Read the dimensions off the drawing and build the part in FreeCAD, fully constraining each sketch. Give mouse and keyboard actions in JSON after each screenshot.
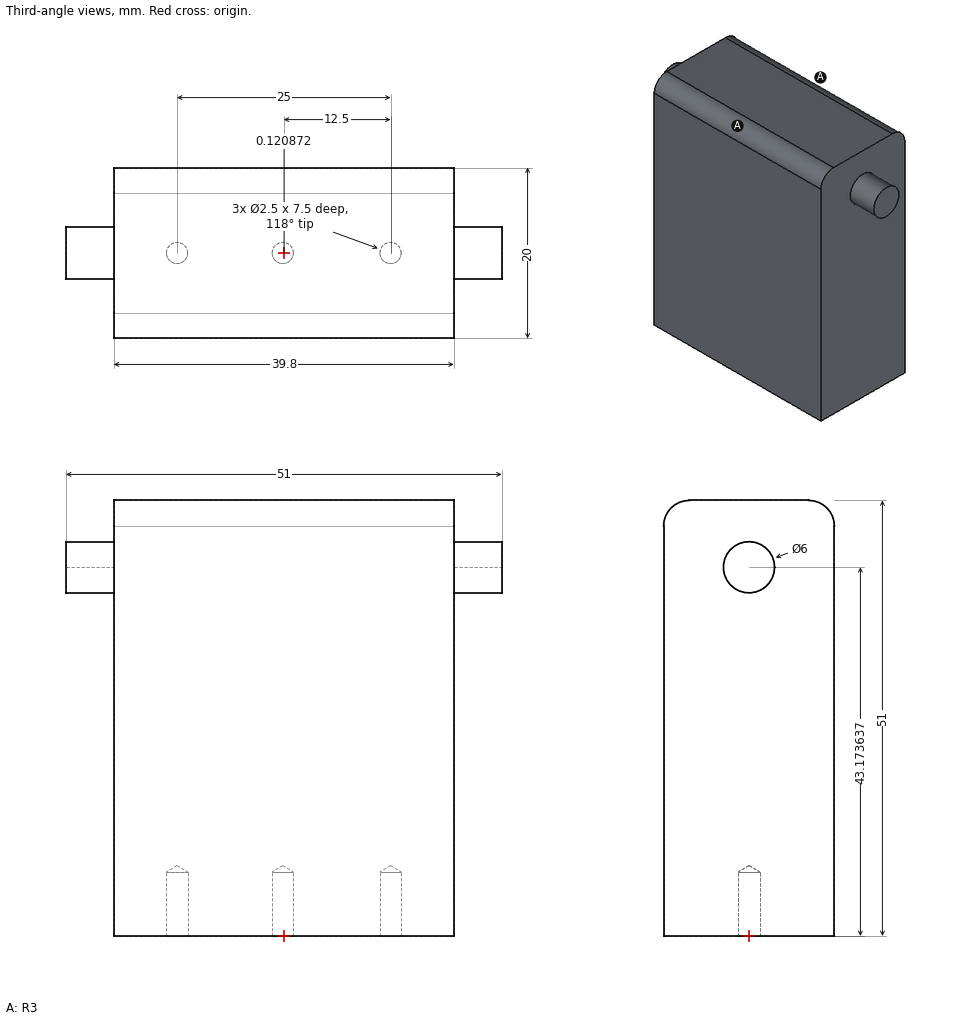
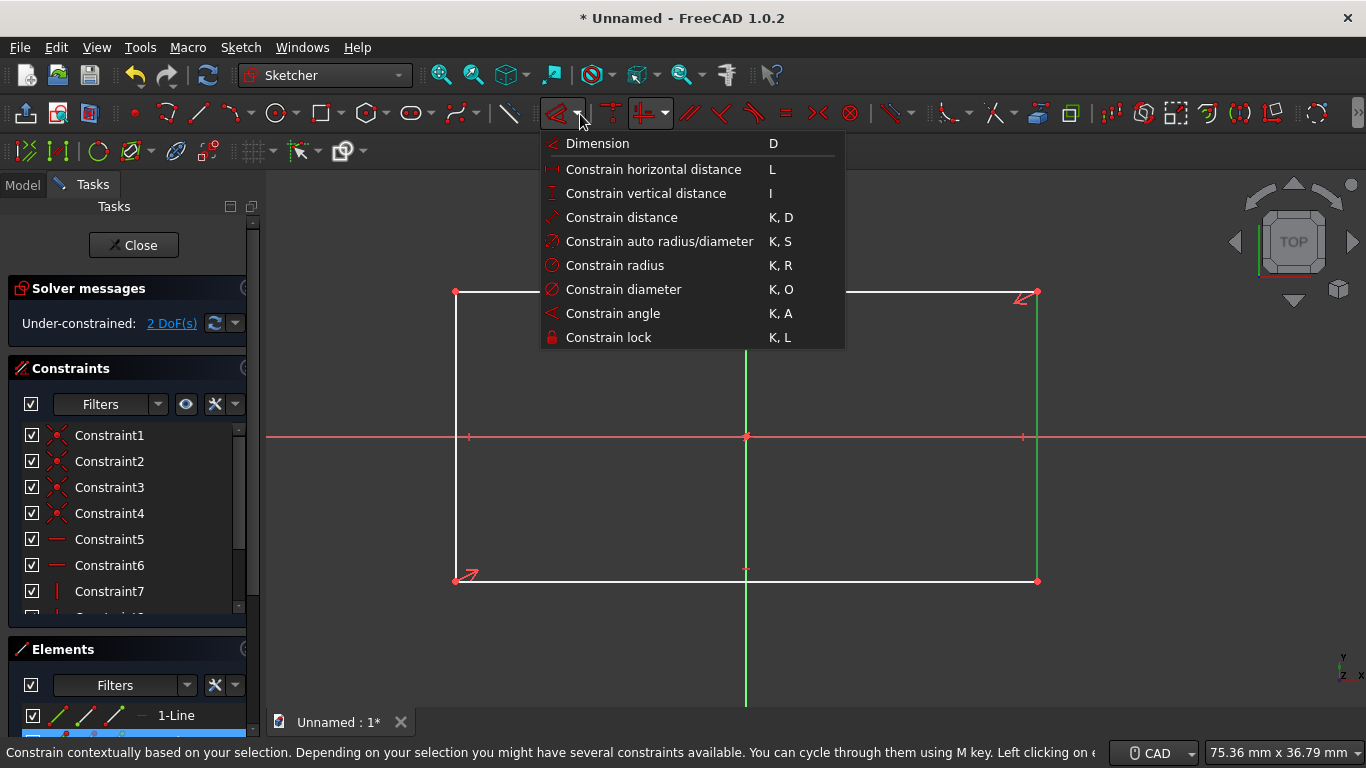
{"action": "left_click", "coordinate": [693, 193]}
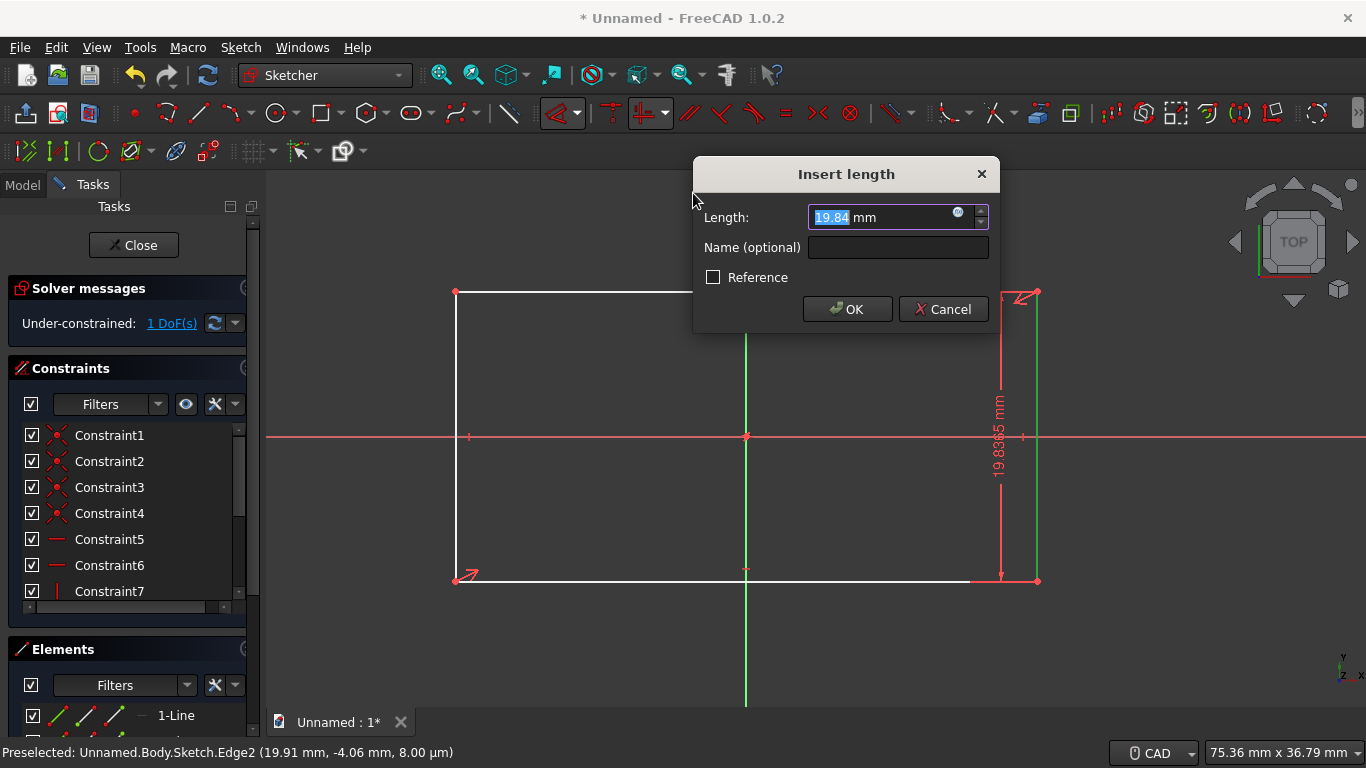
{"action": "type", "text": "20"}
{"action": "key", "text": "Return"}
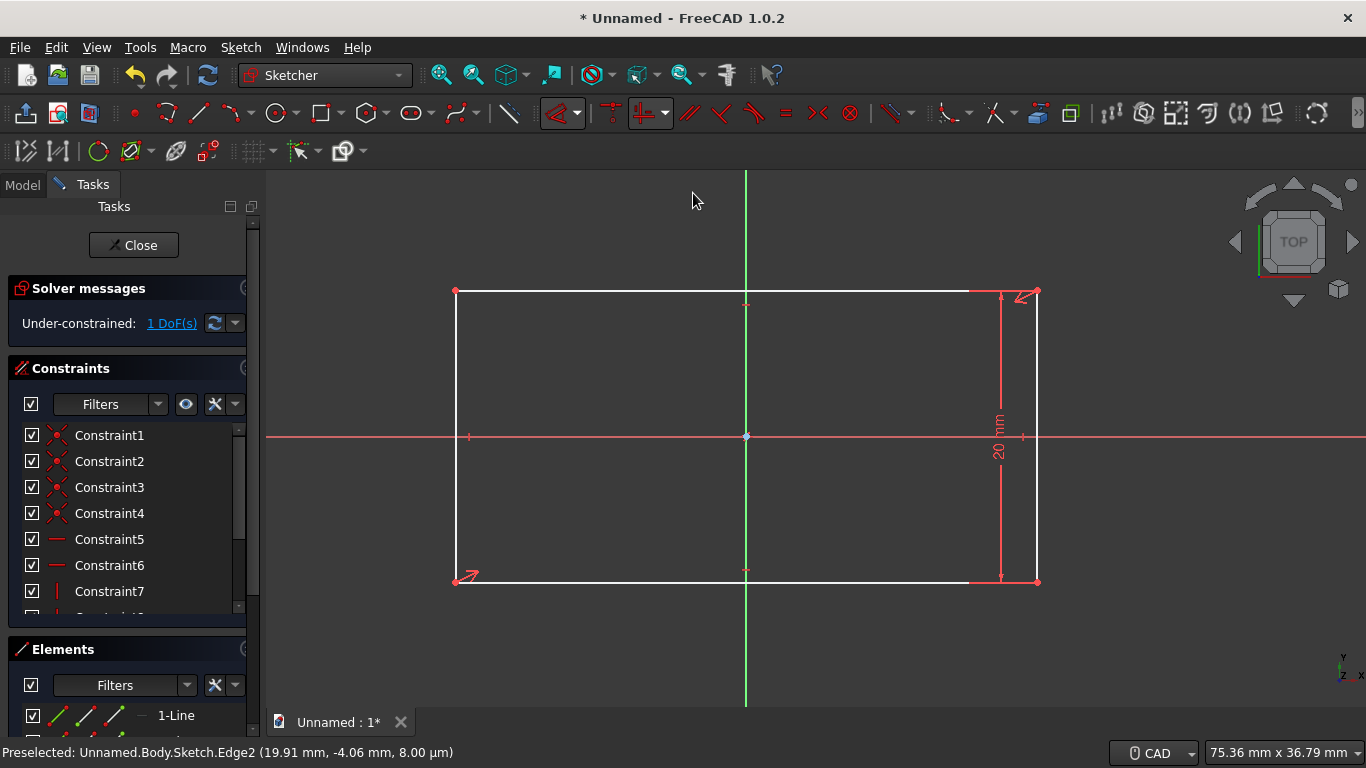
{"action": "left_click", "coordinate": [630, 583]}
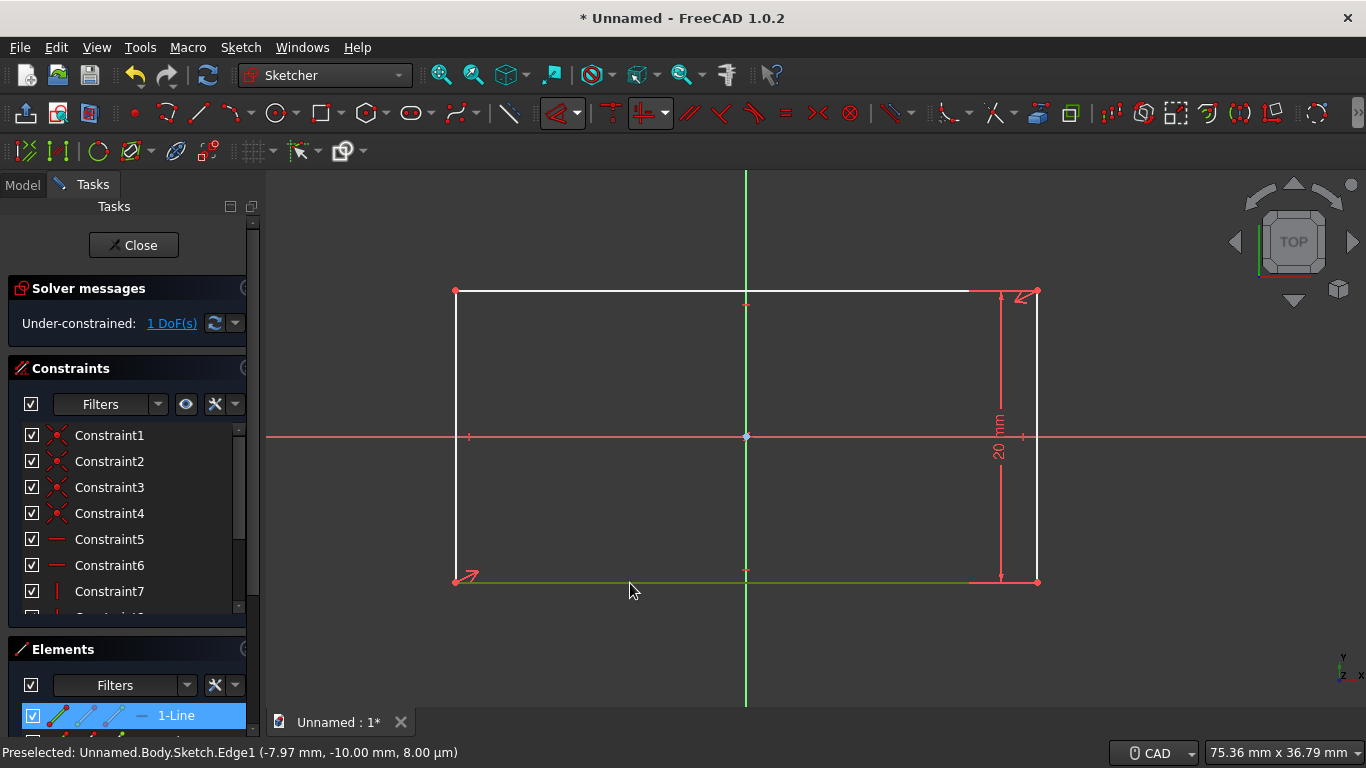
{"action": "key", "text": "l"}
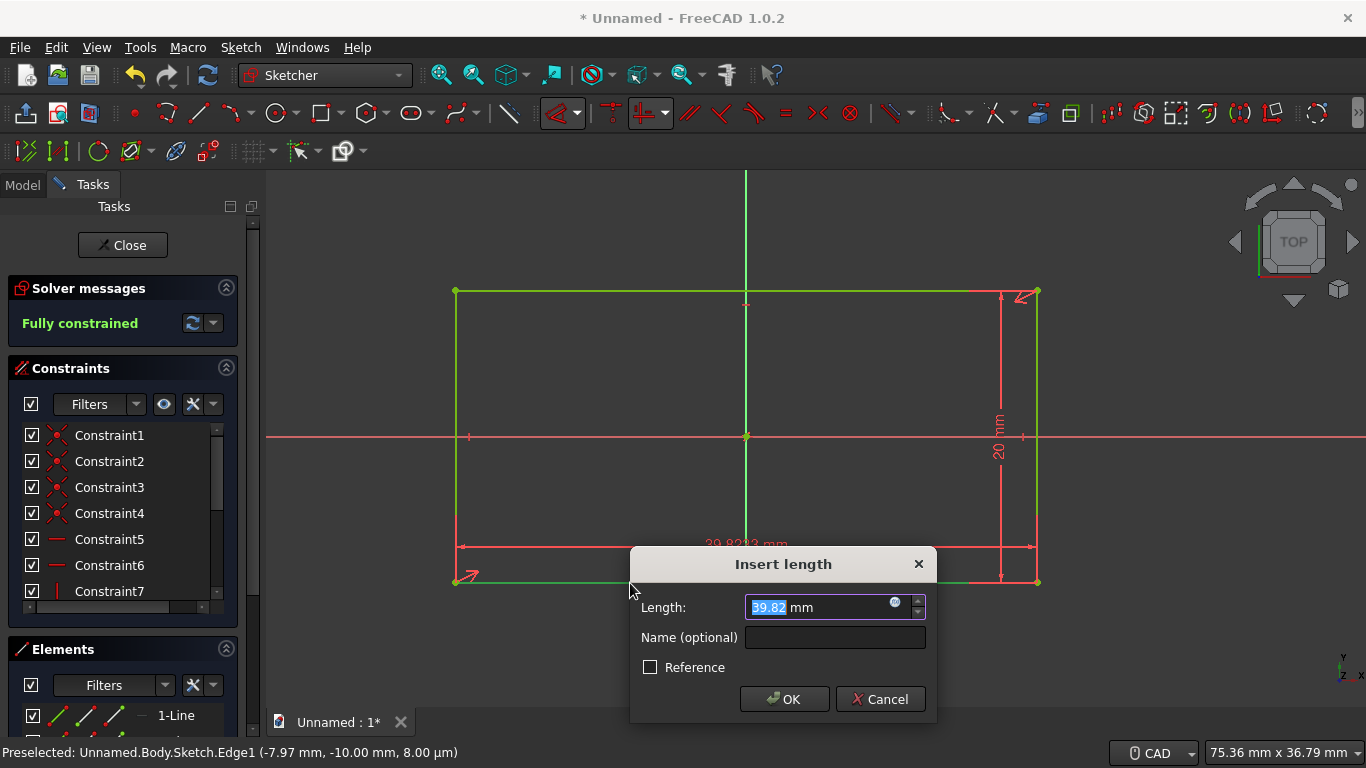
{"action": "type", "text": "39.8"}
{"action": "key", "text": "Return"}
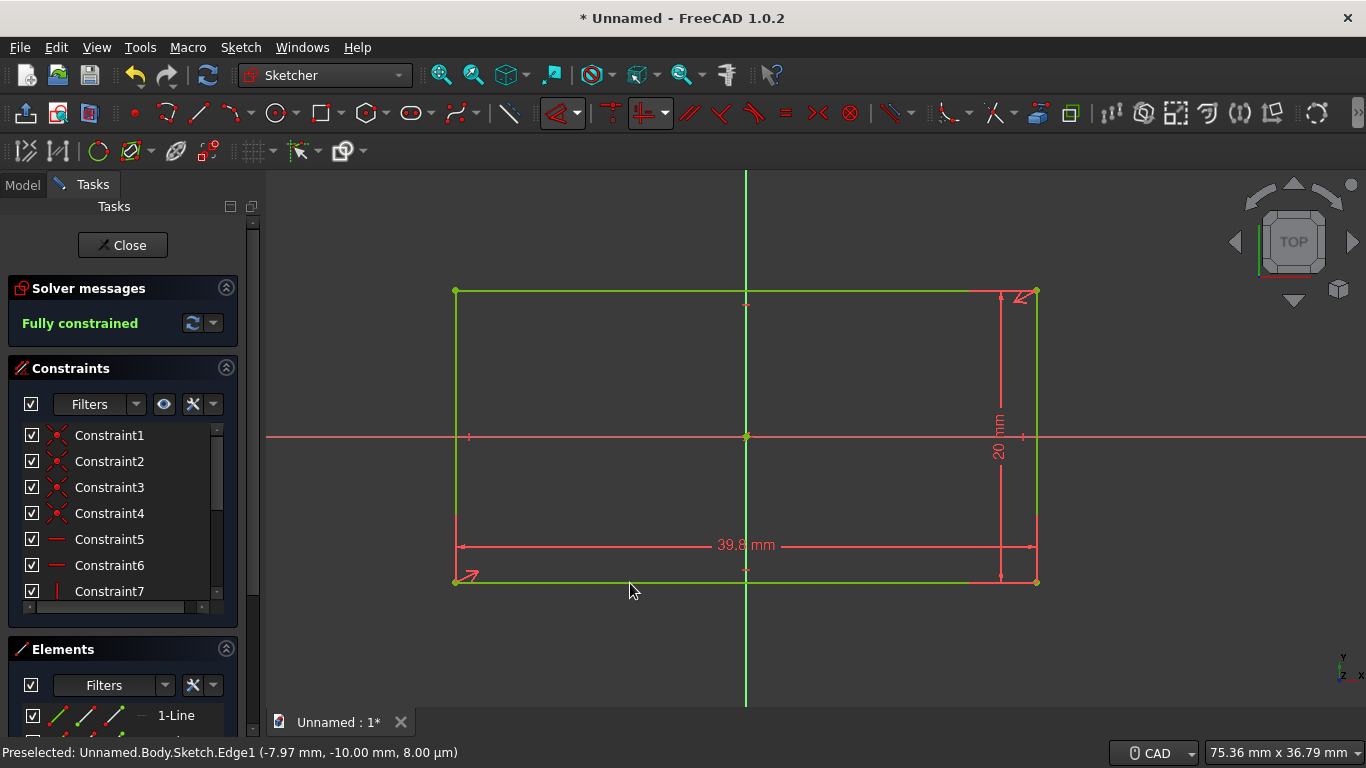
{"action": "left_click", "coordinate": [123, 245]}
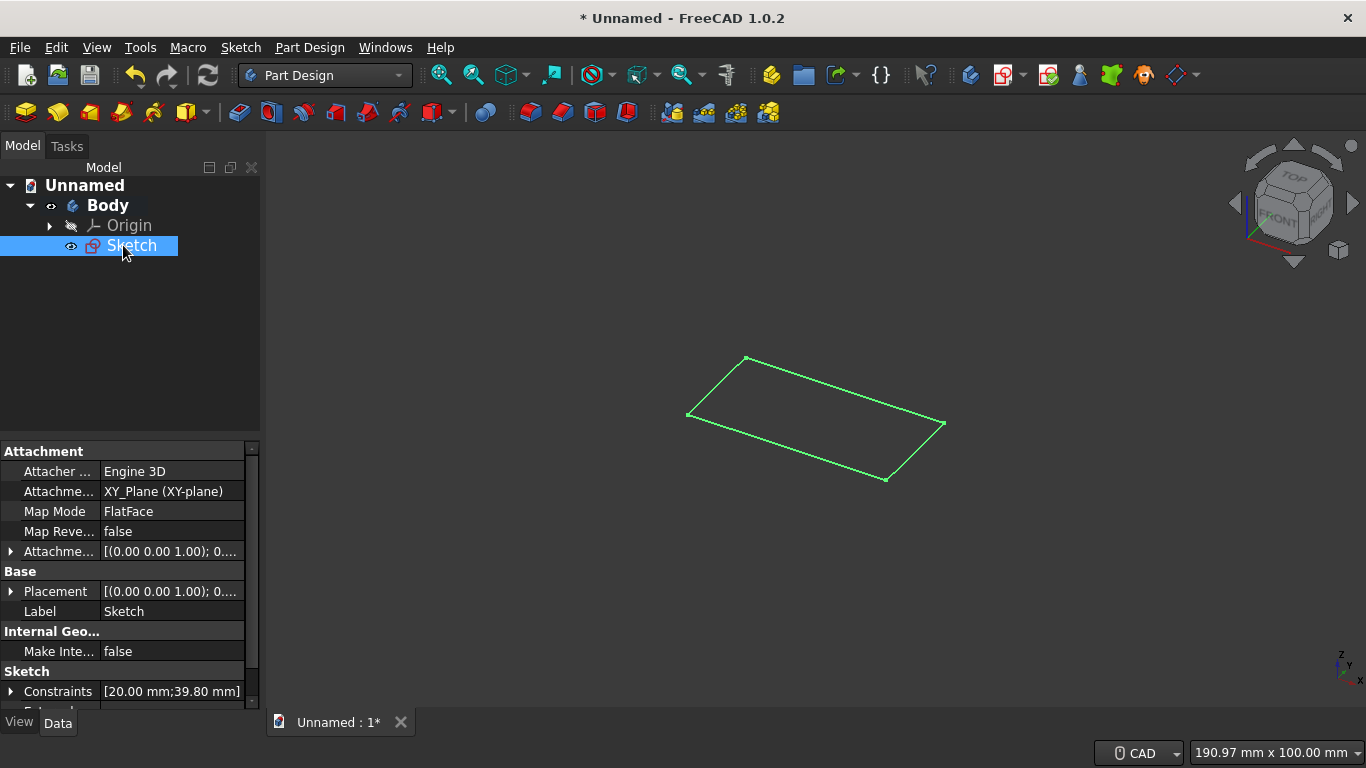
{"action": "left_click", "coordinate": [26, 112]}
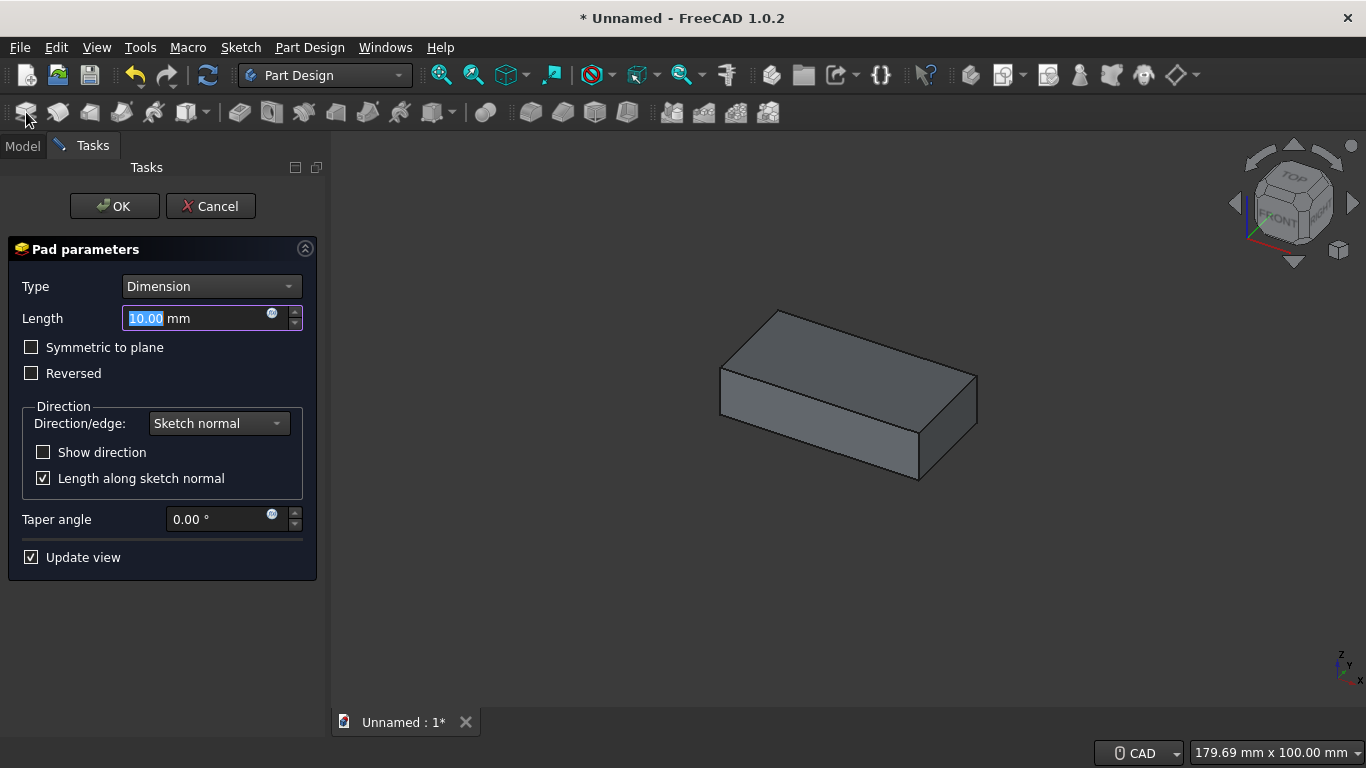
{"action": "type", "text": "51"}
{"action": "key", "text": "Tab"}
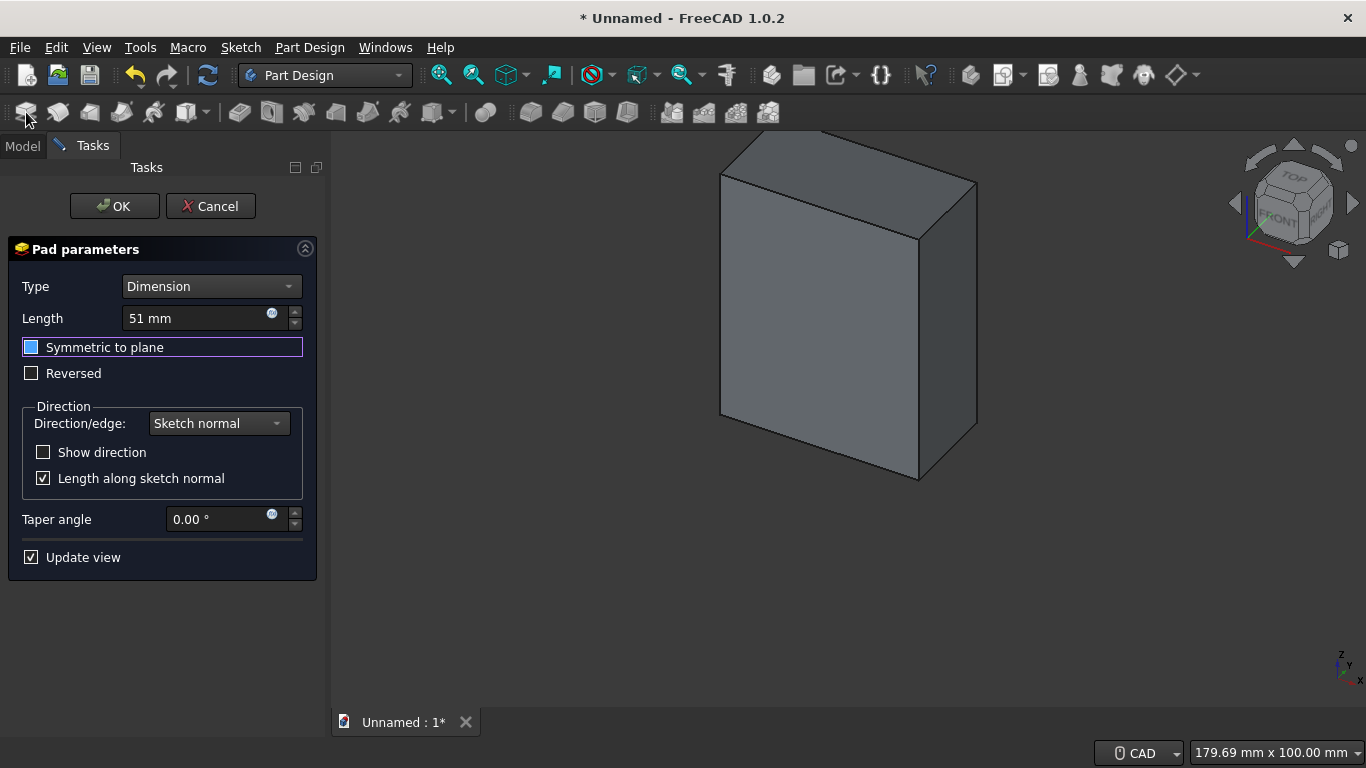
{"action": "left_click", "coordinate": [115, 206]}